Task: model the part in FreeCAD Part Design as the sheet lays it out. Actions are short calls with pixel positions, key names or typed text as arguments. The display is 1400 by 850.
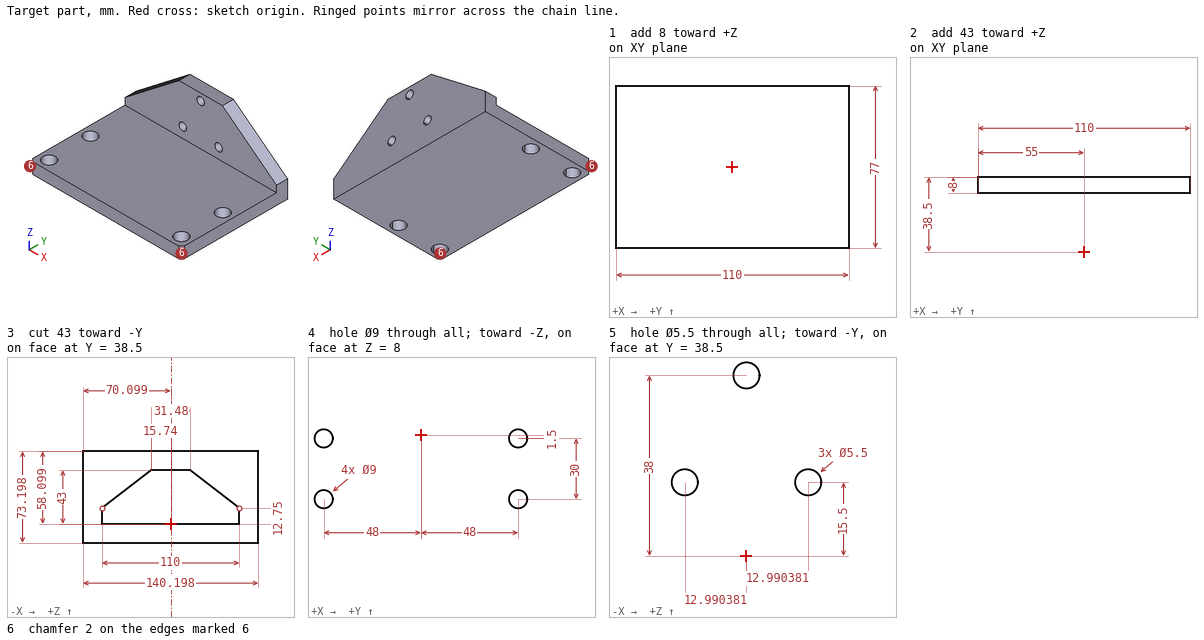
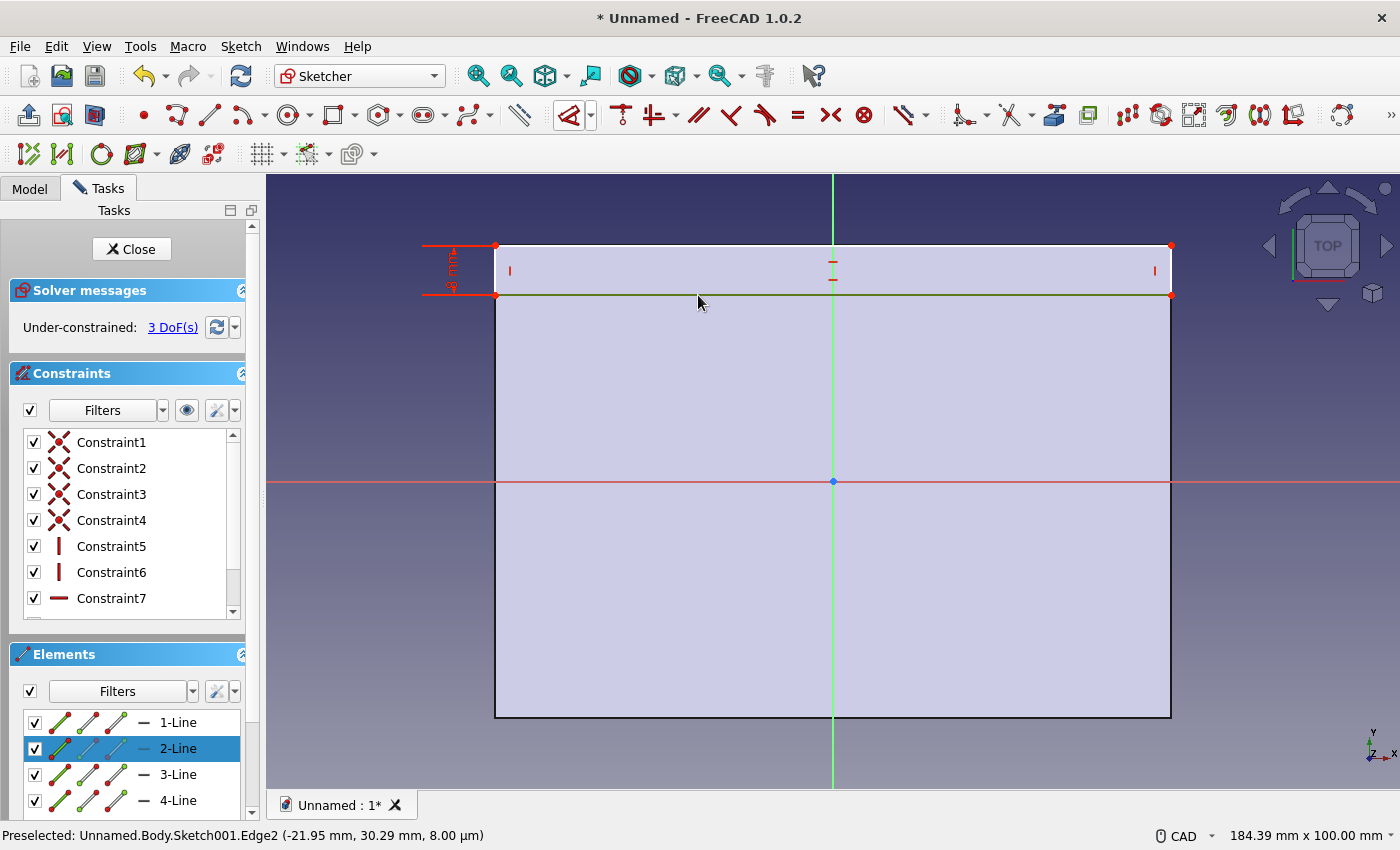
key(l)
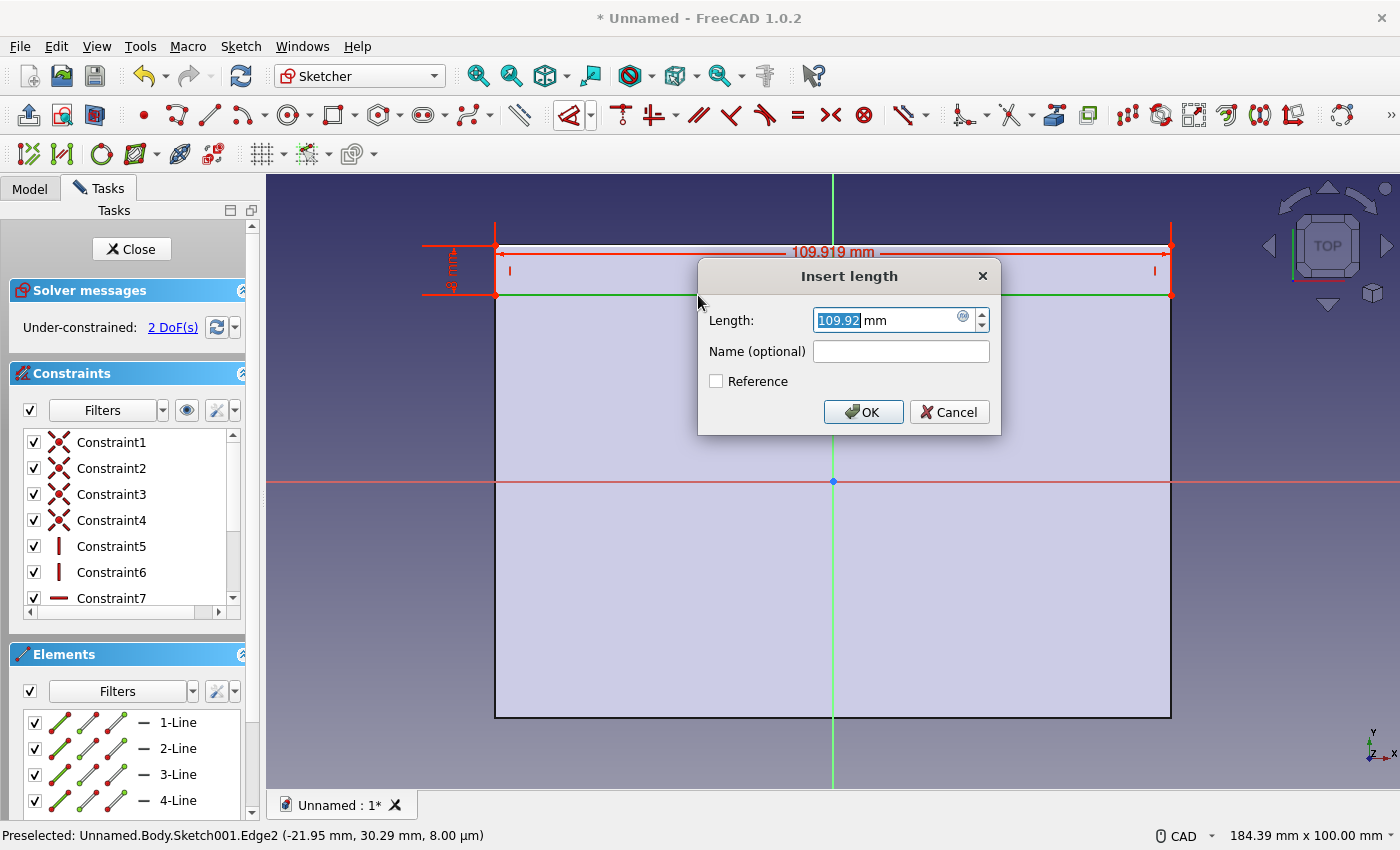
text(110)
key(Return)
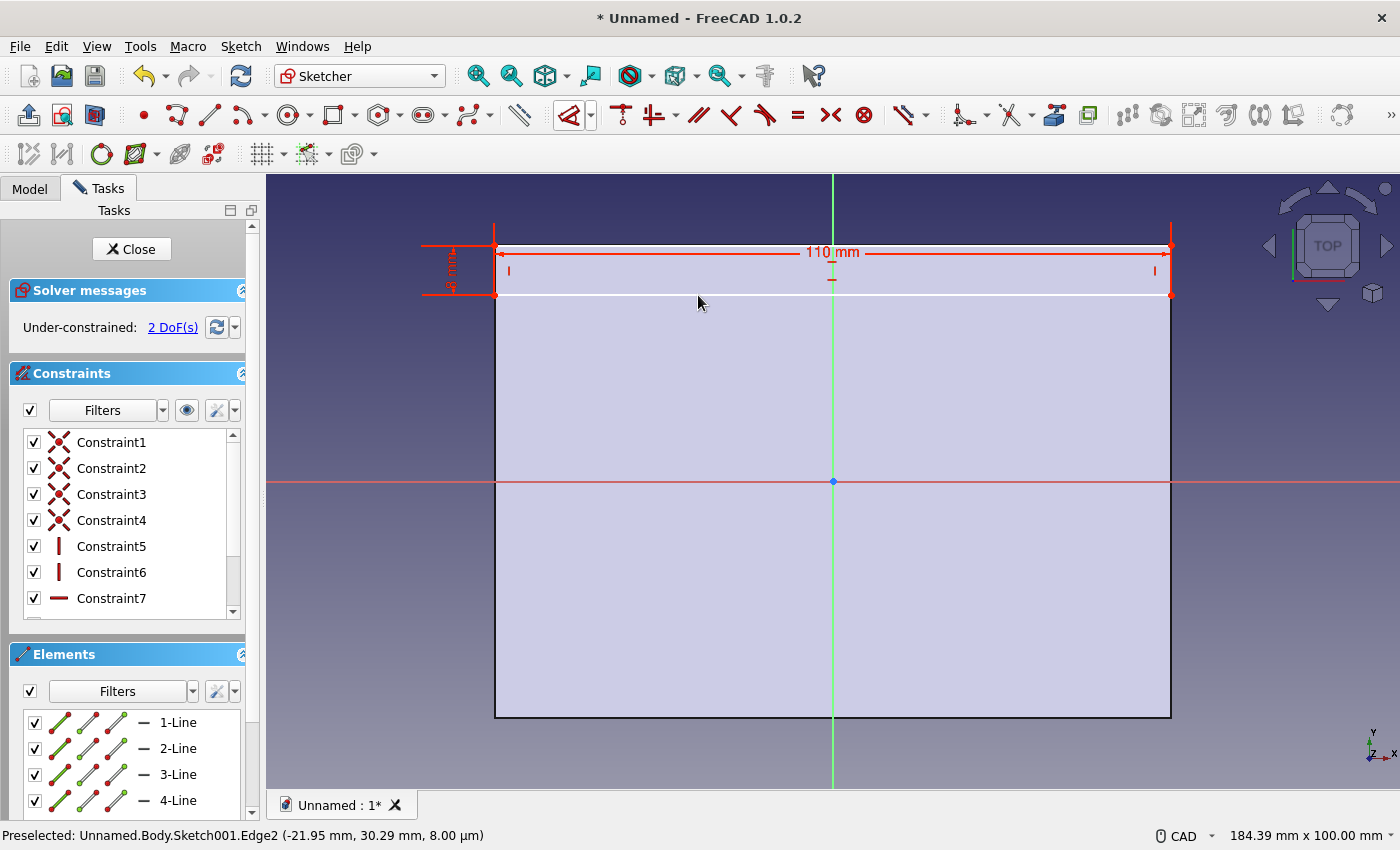
click(494, 246)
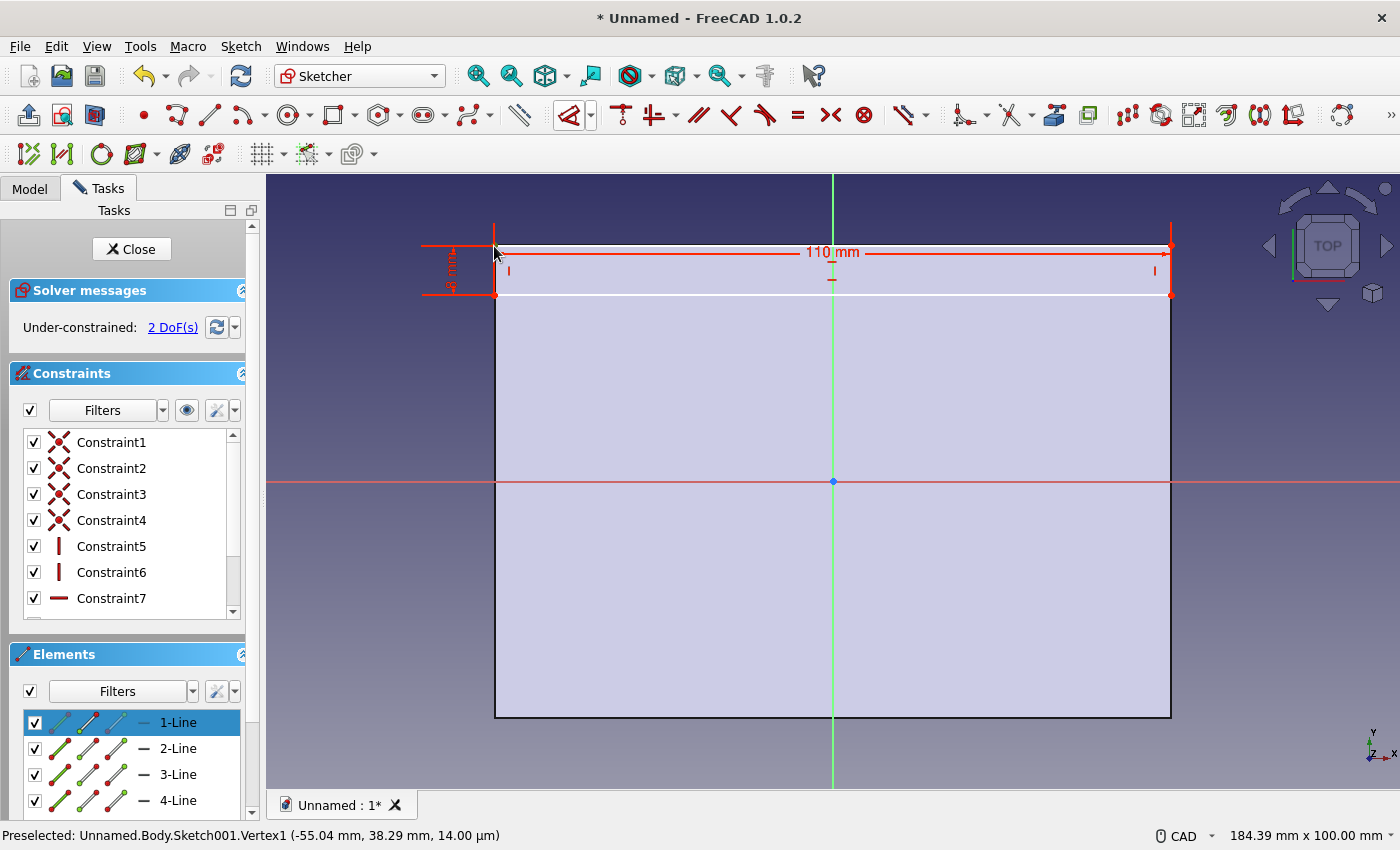
key(l)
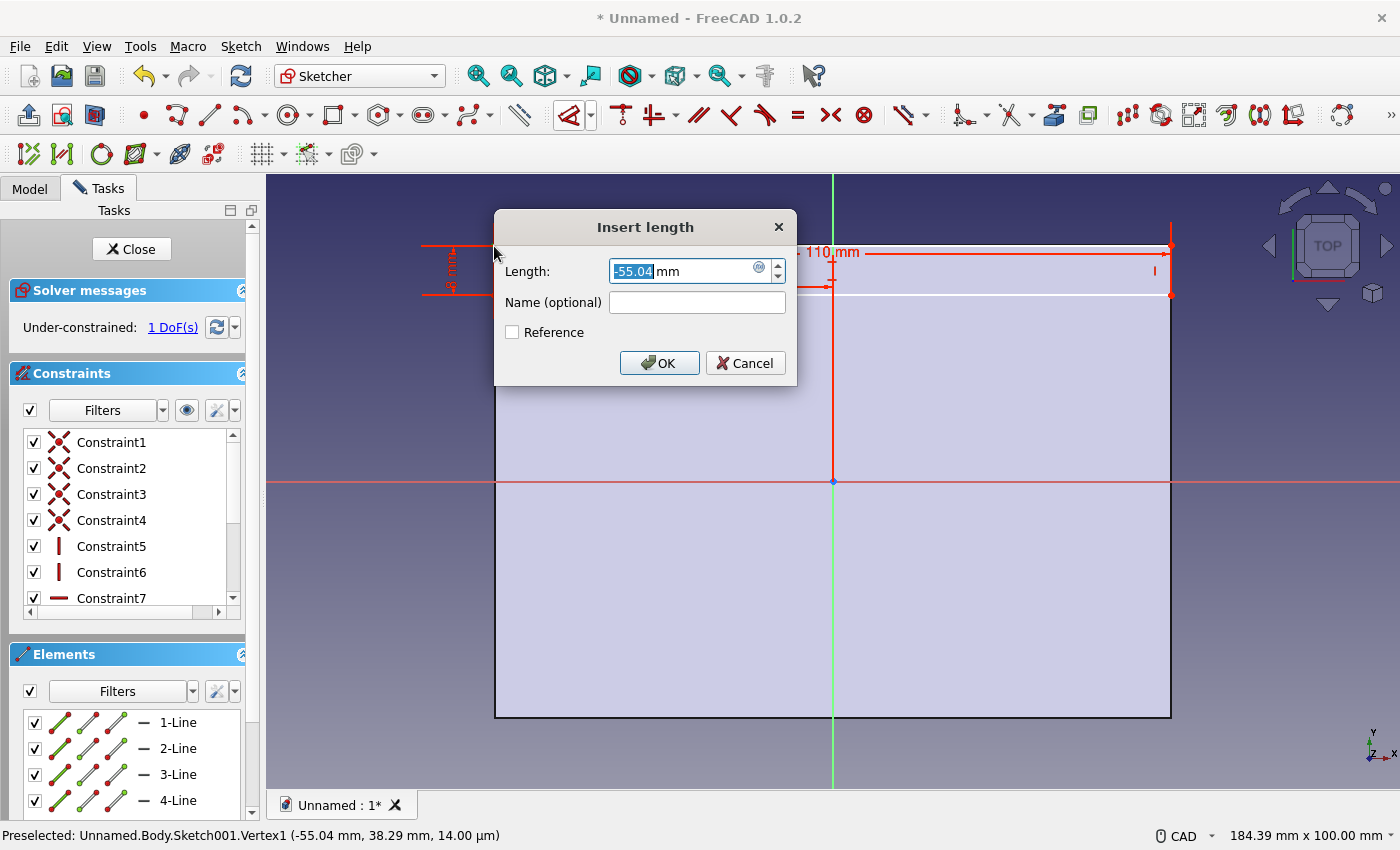
text(-55)
key(Return)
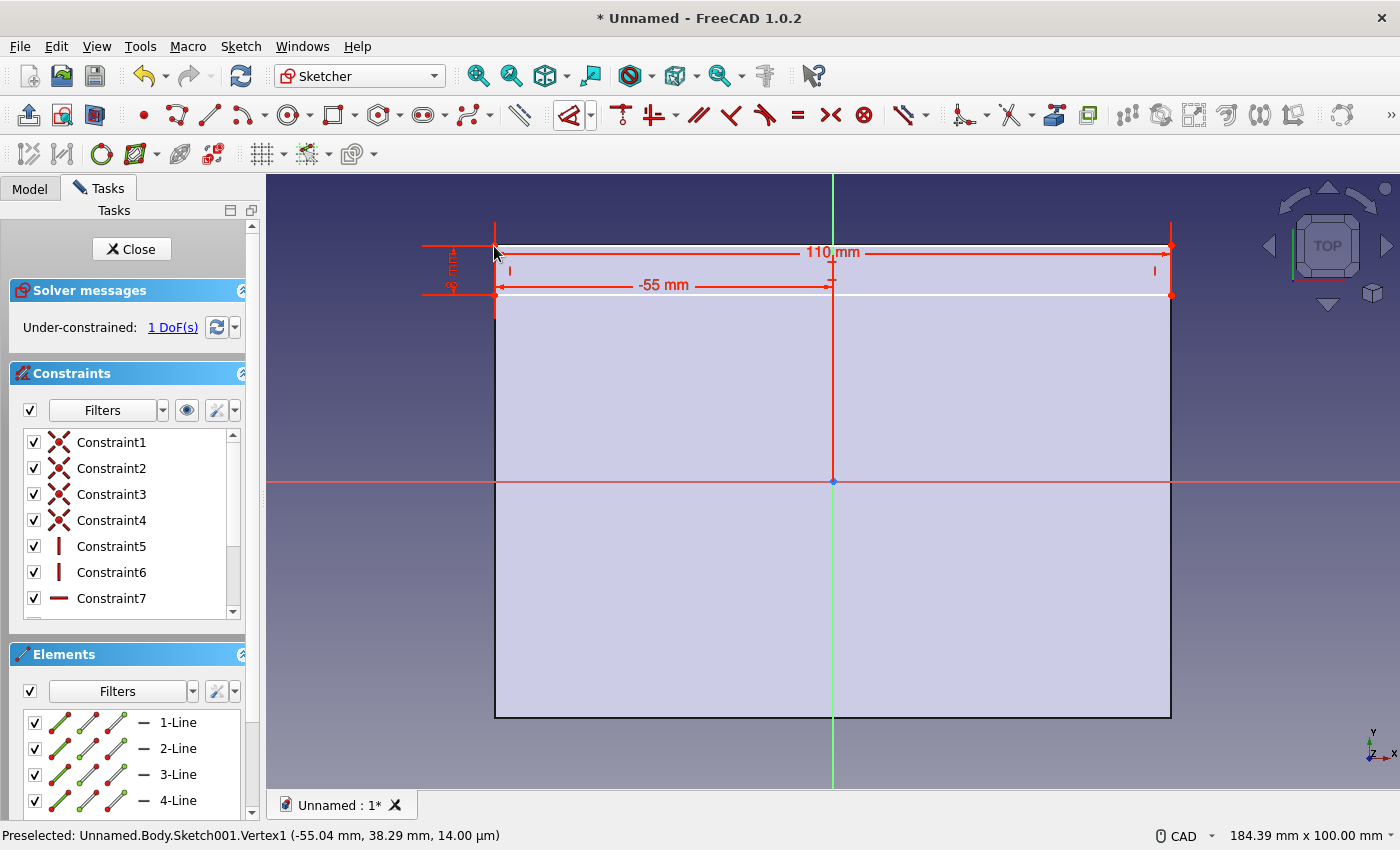
click(495, 246)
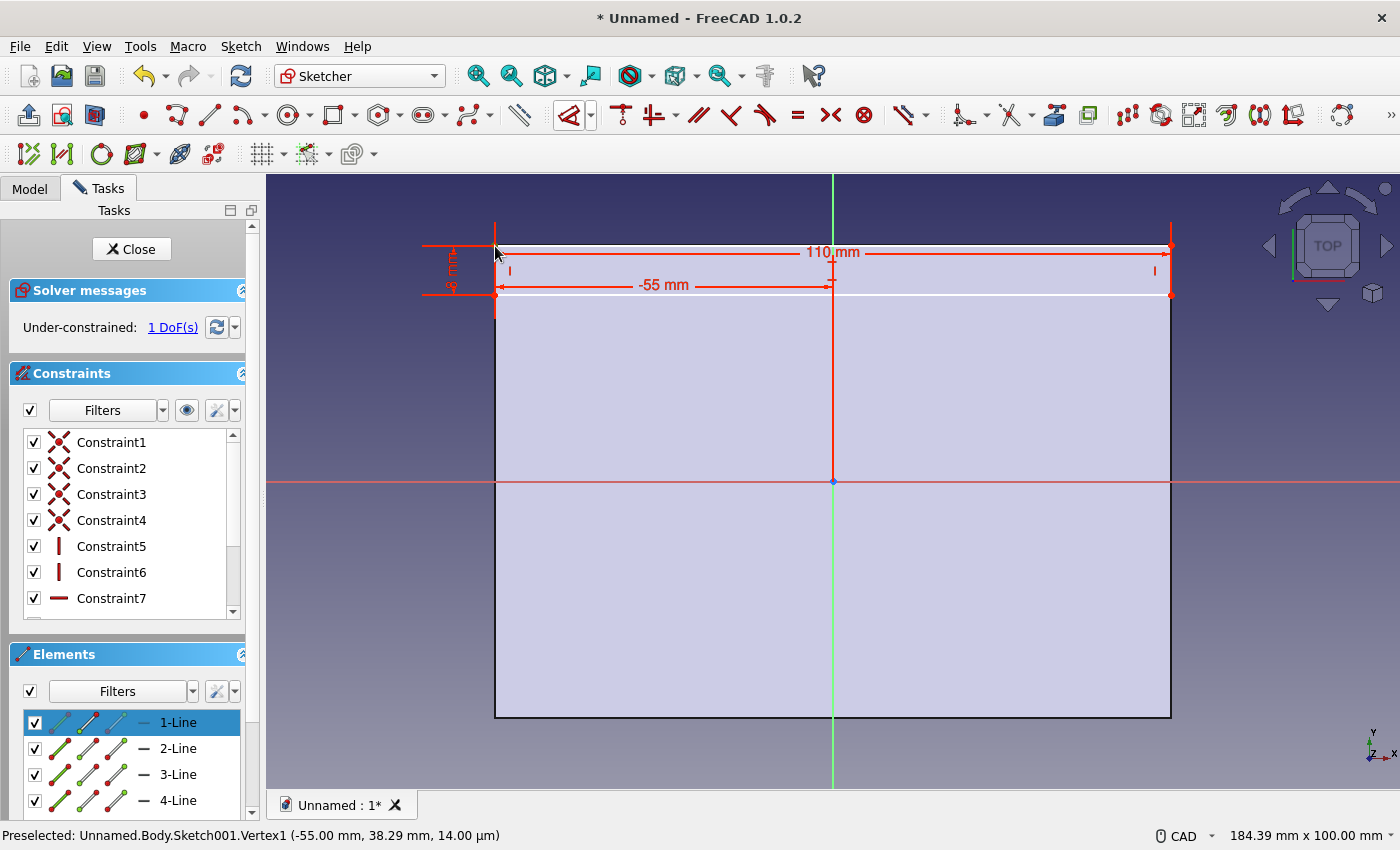
key(i)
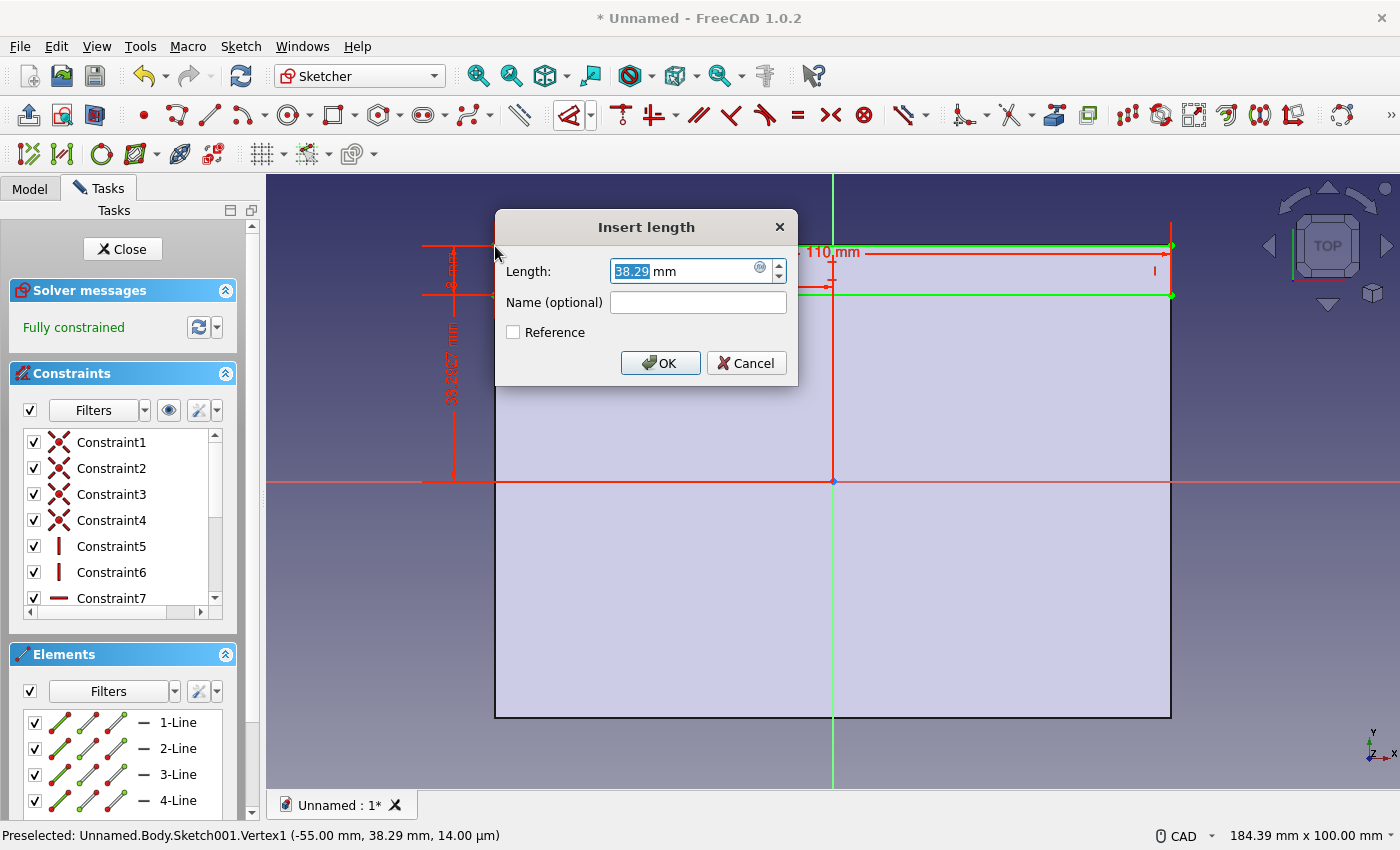
text(38.5)
key(Return)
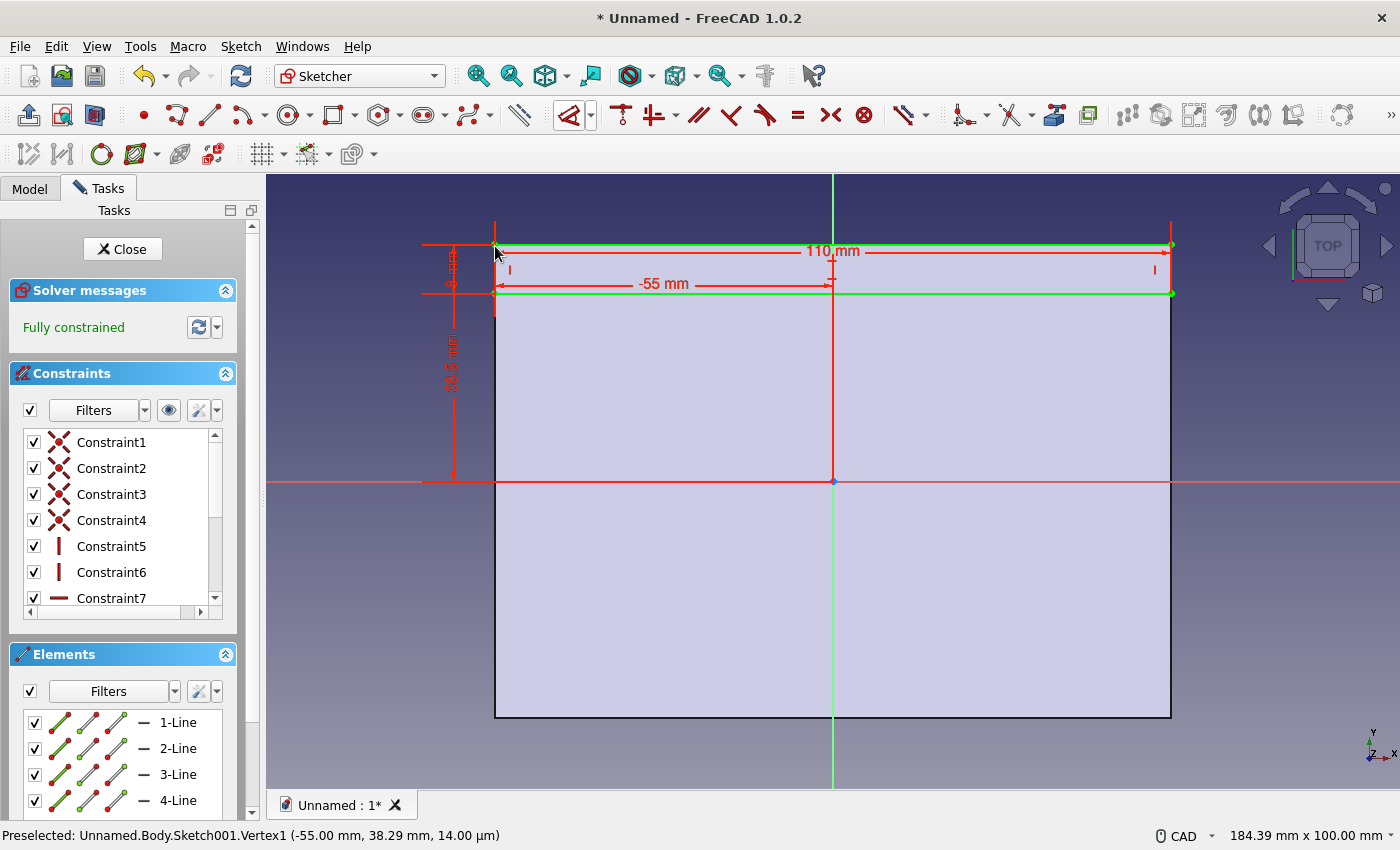
click(123, 249)